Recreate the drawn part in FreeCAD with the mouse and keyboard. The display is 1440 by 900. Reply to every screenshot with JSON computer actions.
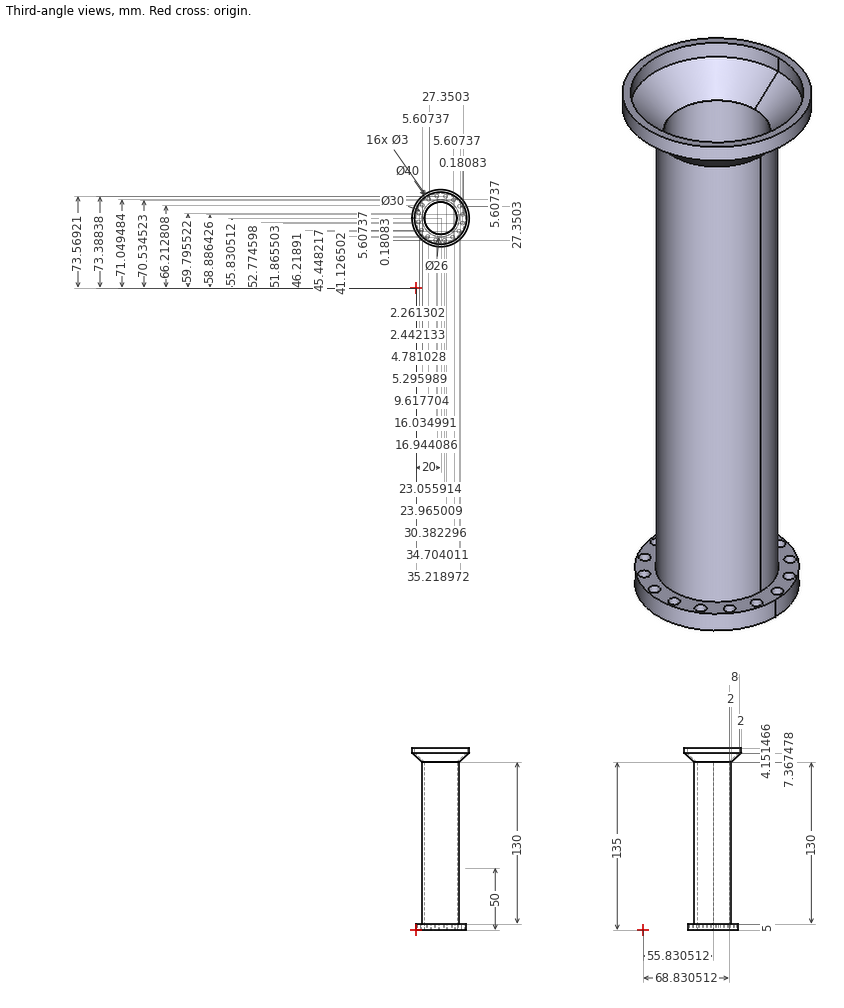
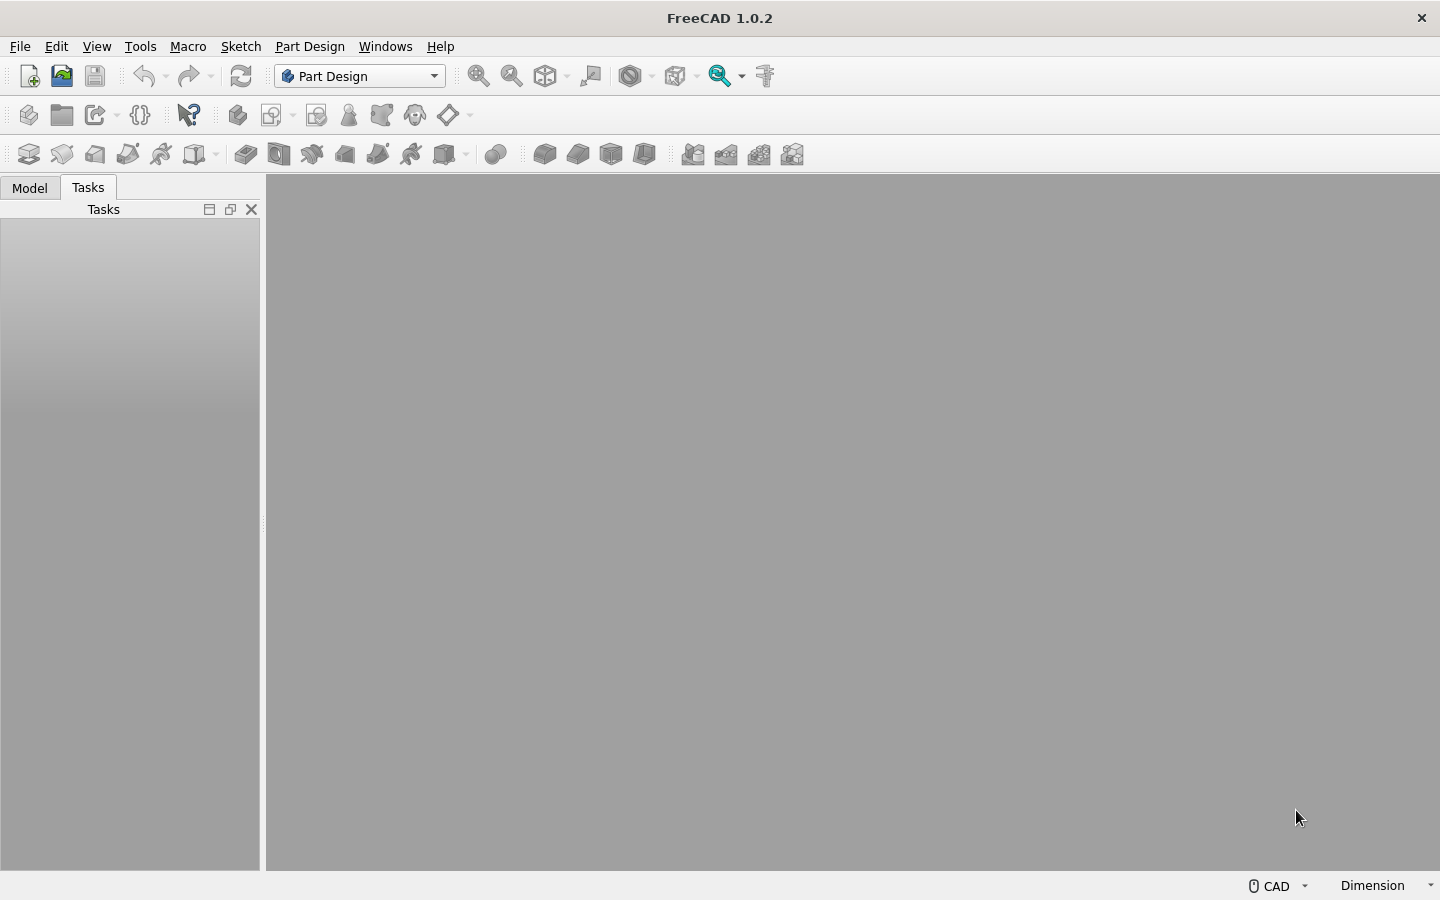
{"action": "left_click", "coordinate": [29, 76]}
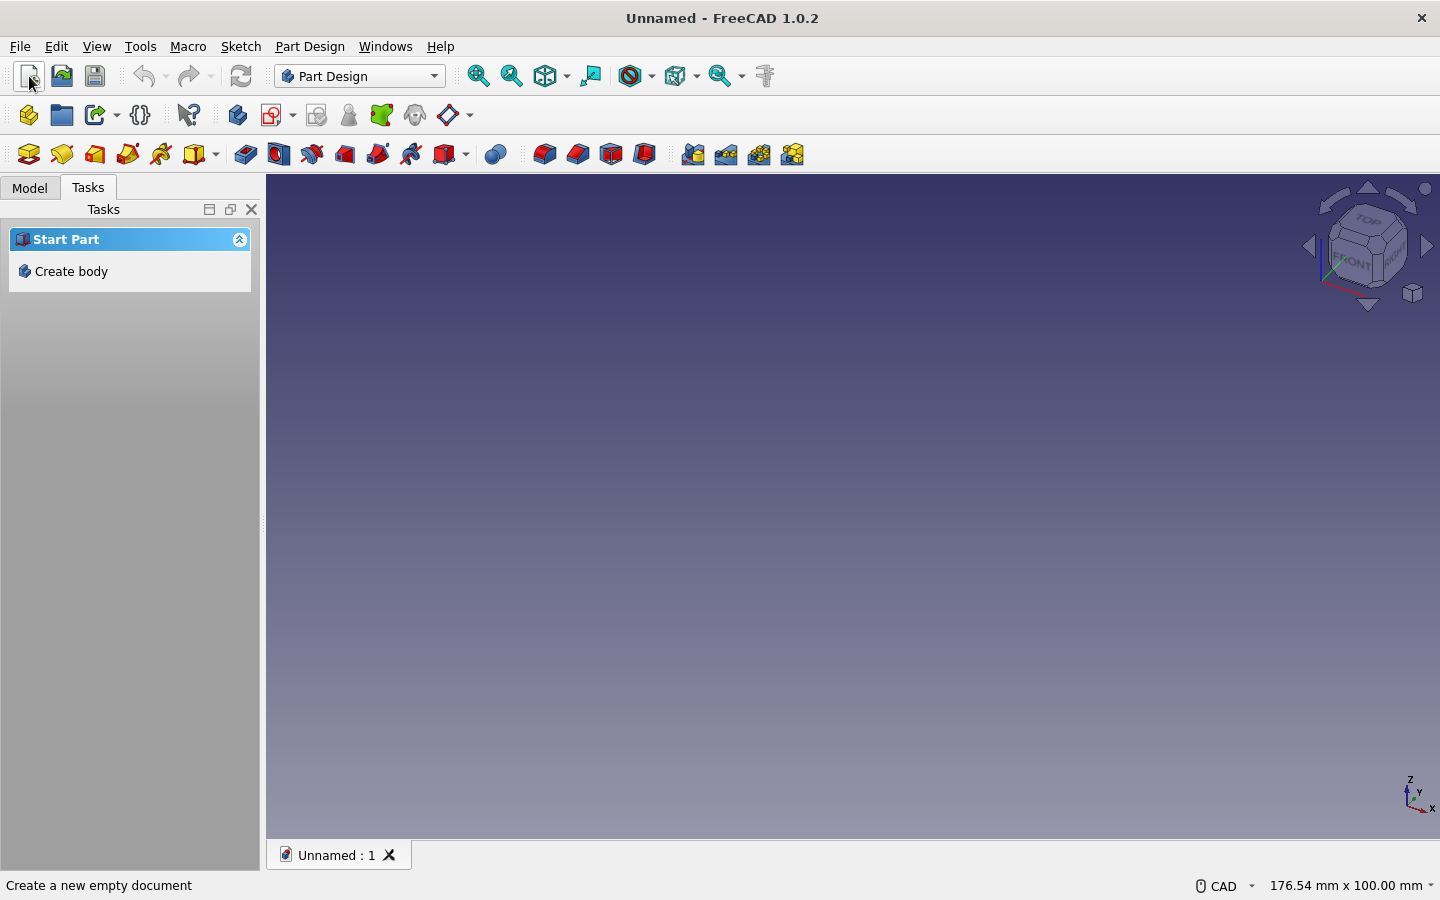
{"action": "left_click", "coordinate": [270, 116]}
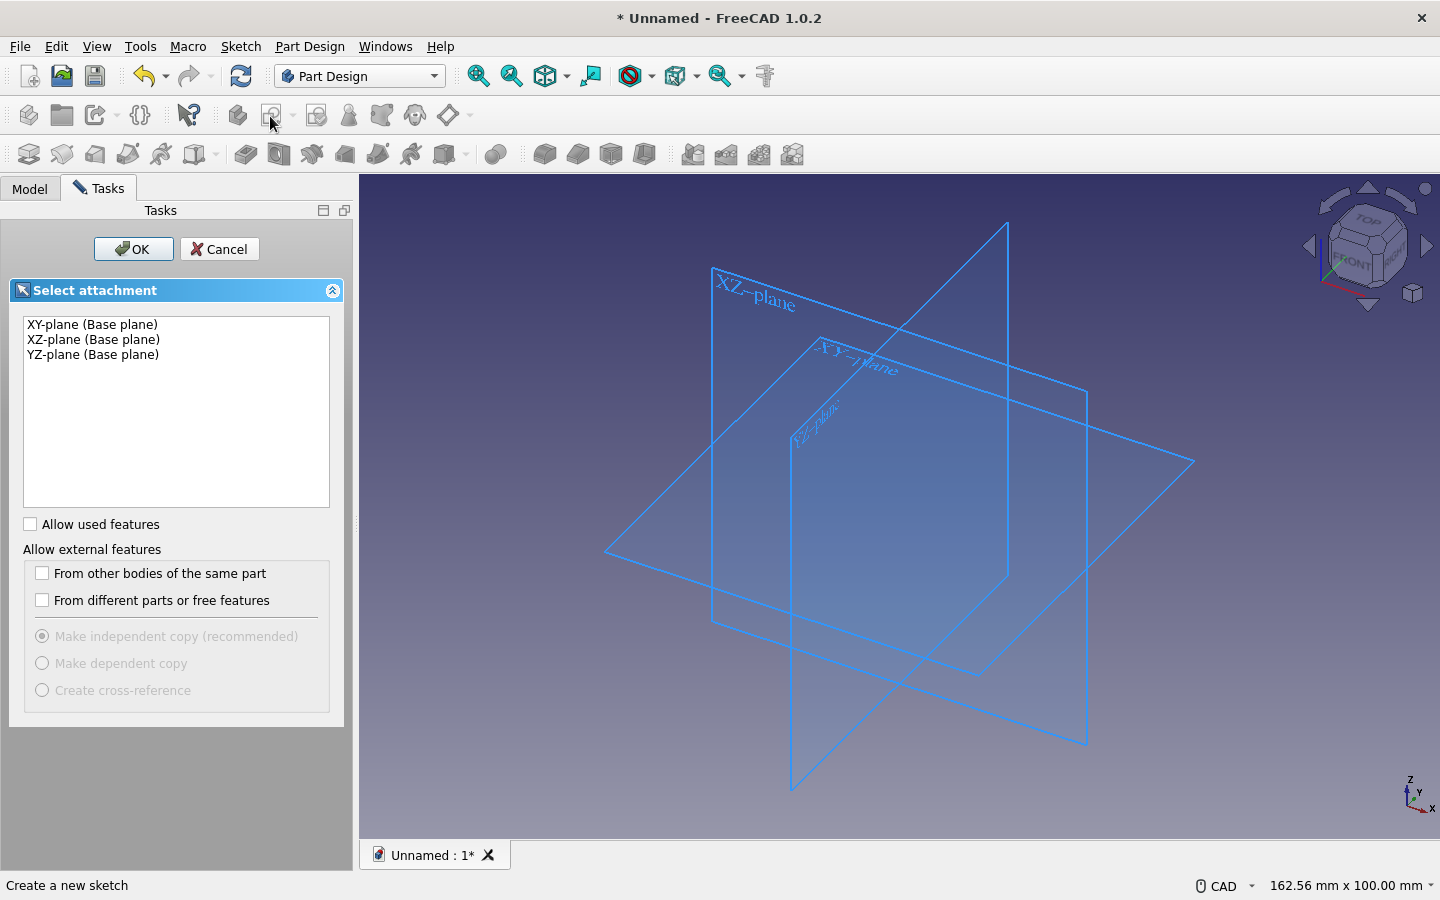
{"action": "left_click", "coordinate": [84, 324]}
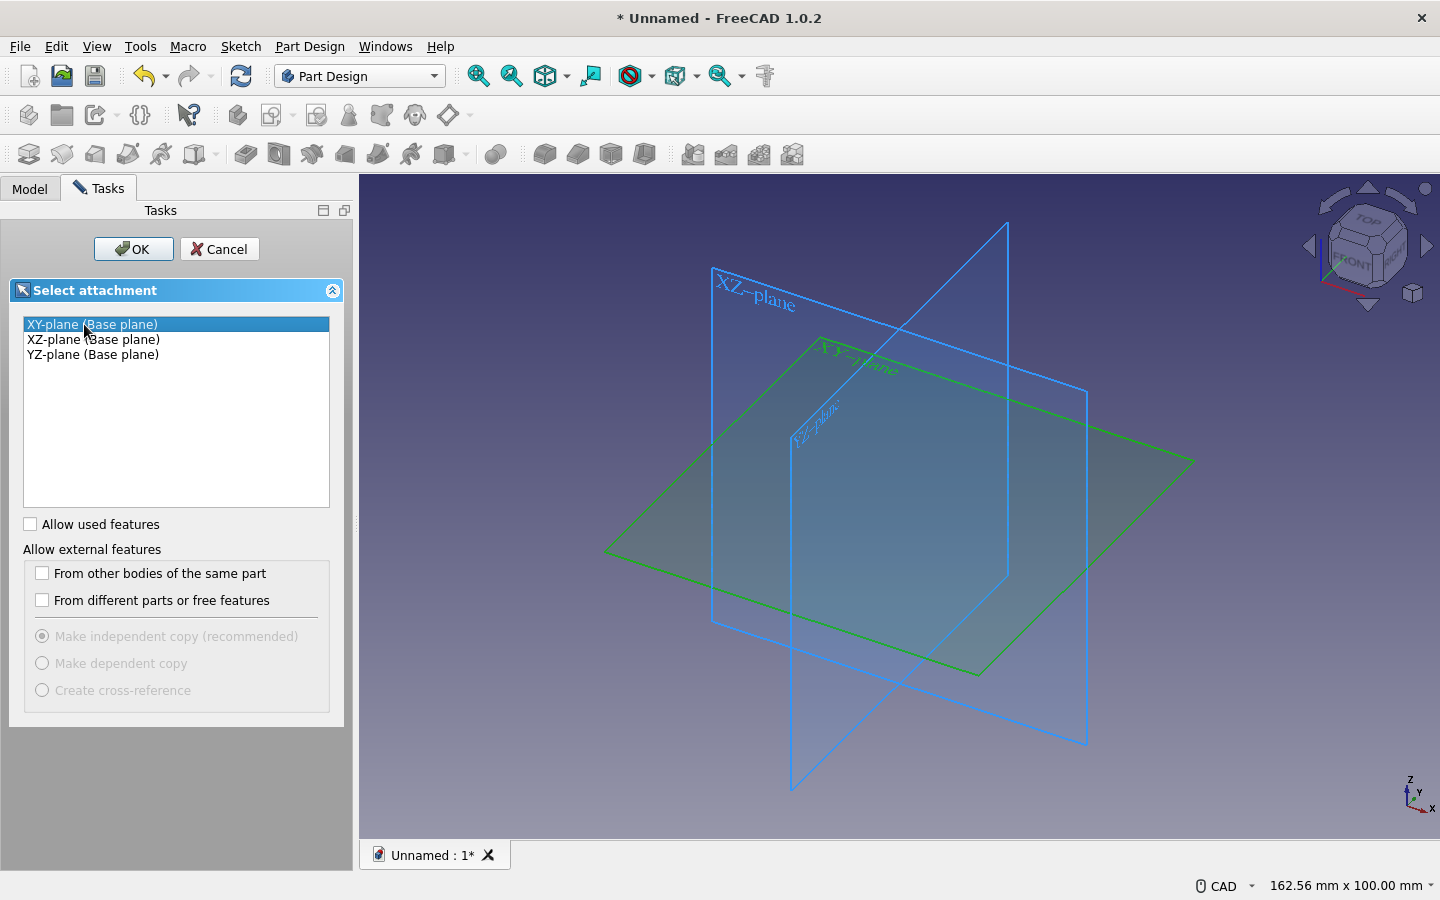
{"action": "left_click", "coordinate": [134, 249]}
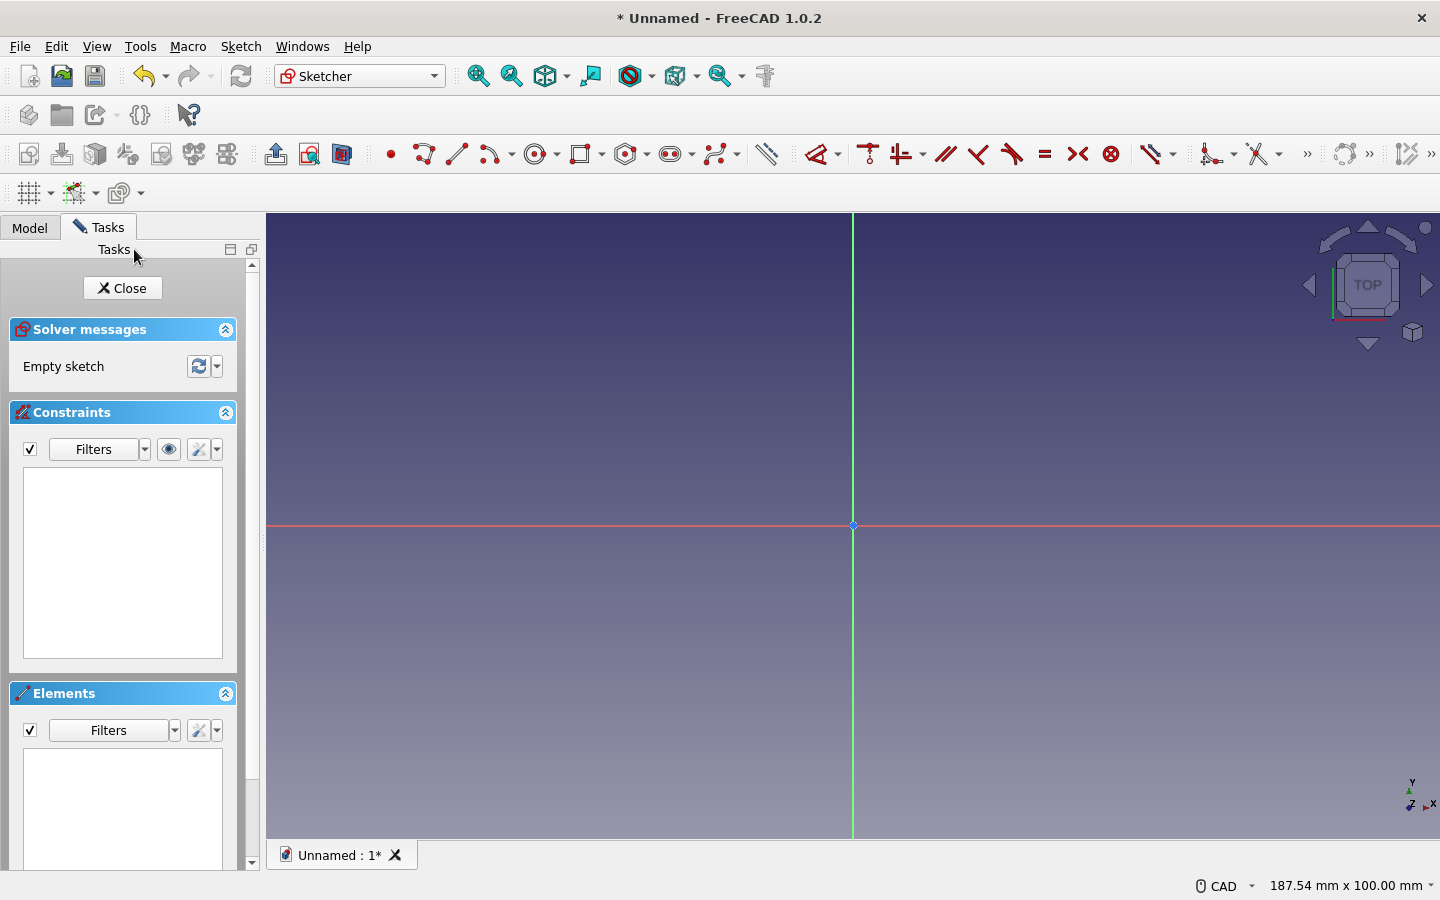
{"action": "scroll", "coordinate": [391, 811], "scroll_direction": "down", "scroll_amount": 2}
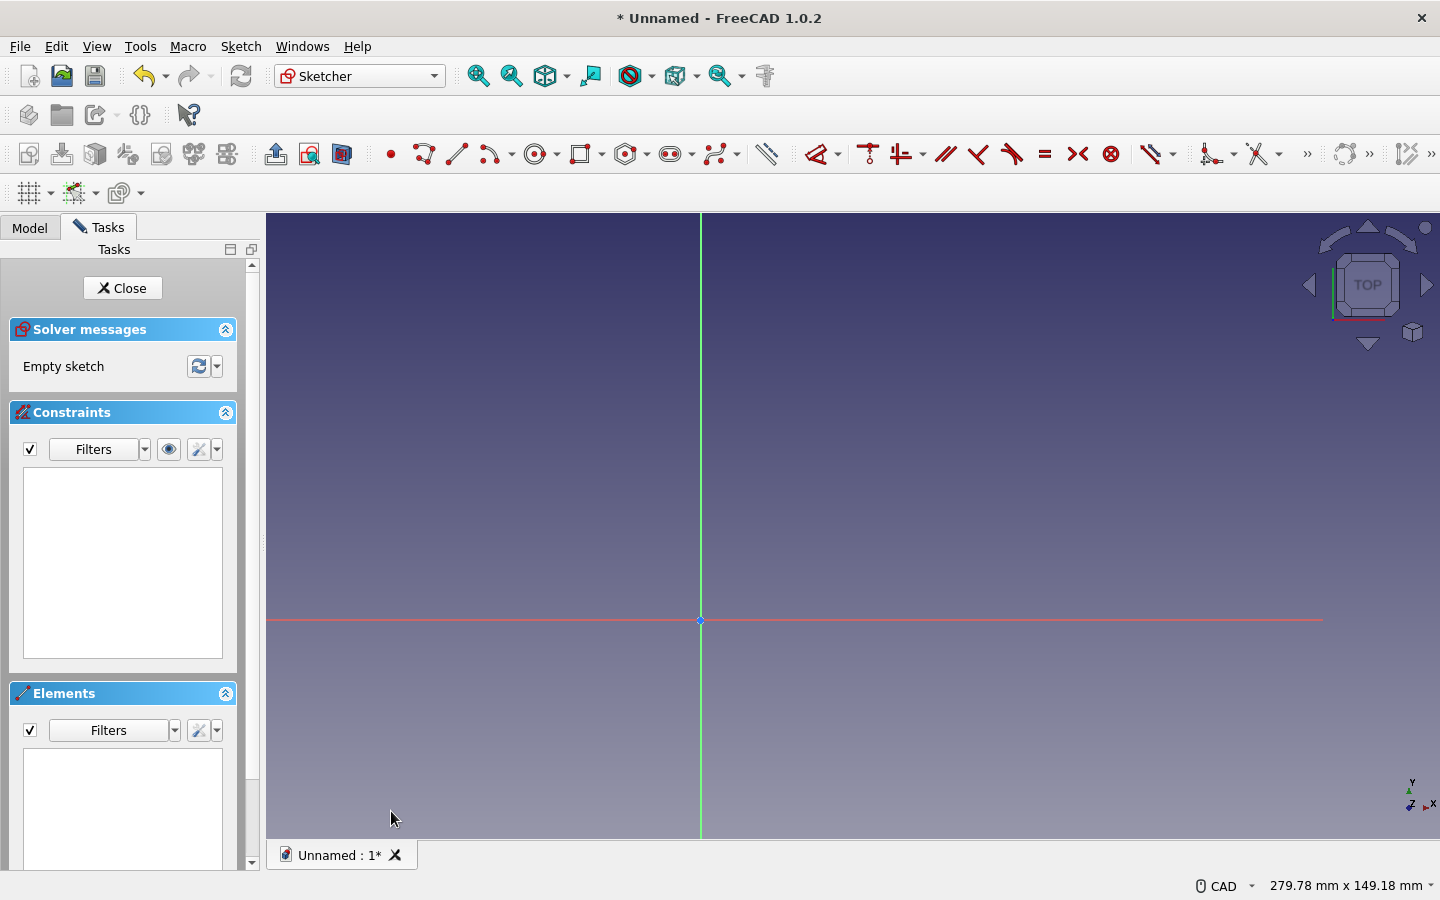
{"action": "left_click", "coordinate": [534, 154]}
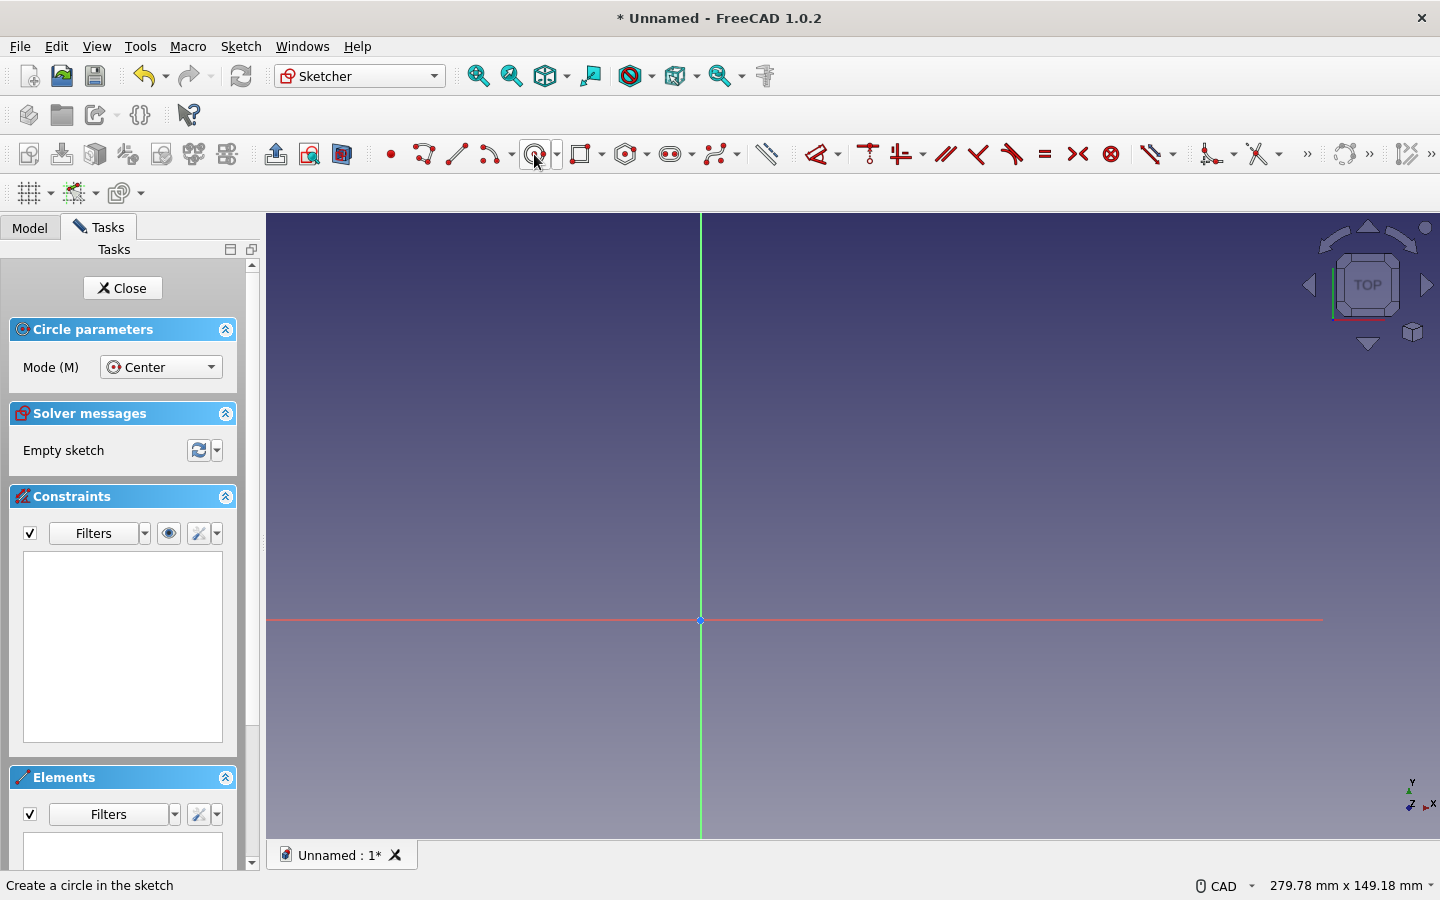
{"action": "left_click", "coordinate": [785, 386]}
{"action": "mouse_move", "coordinate": [844, 327]}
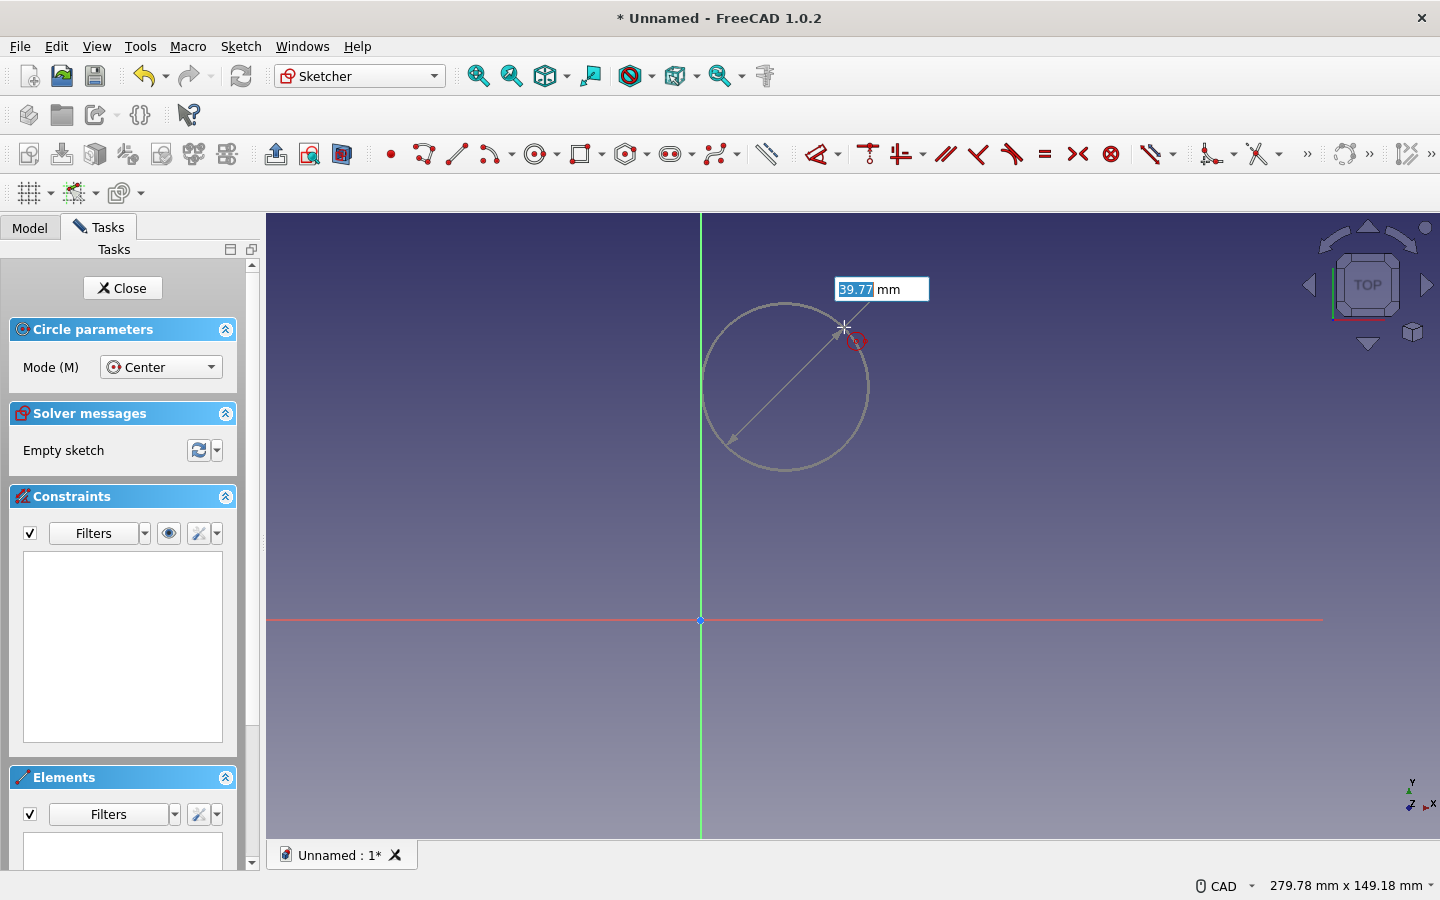
{"action": "type", "text": "40"}
{"action": "key", "text": "Return"}
{"action": "key", "text": "Escape"}